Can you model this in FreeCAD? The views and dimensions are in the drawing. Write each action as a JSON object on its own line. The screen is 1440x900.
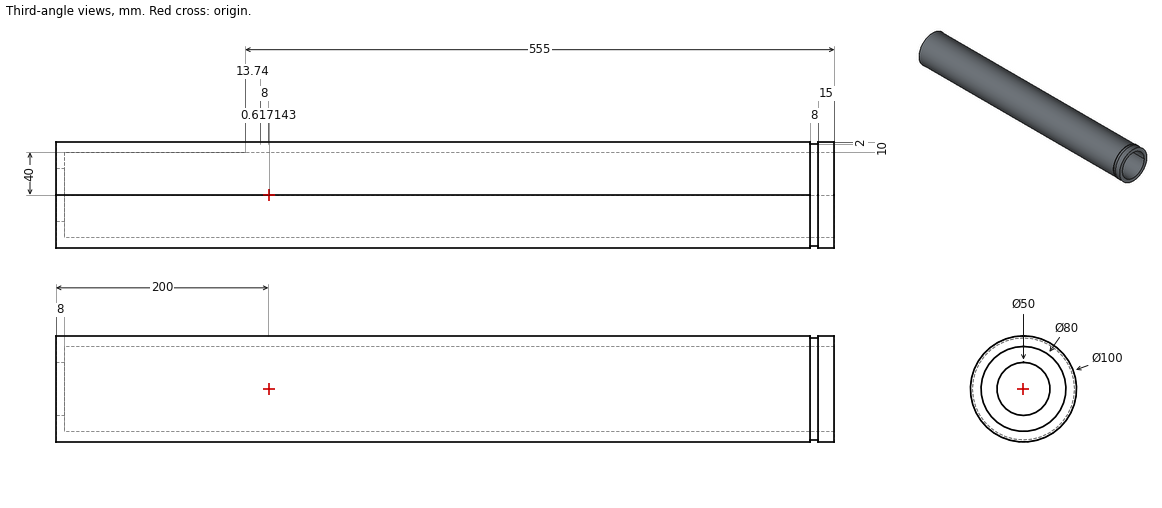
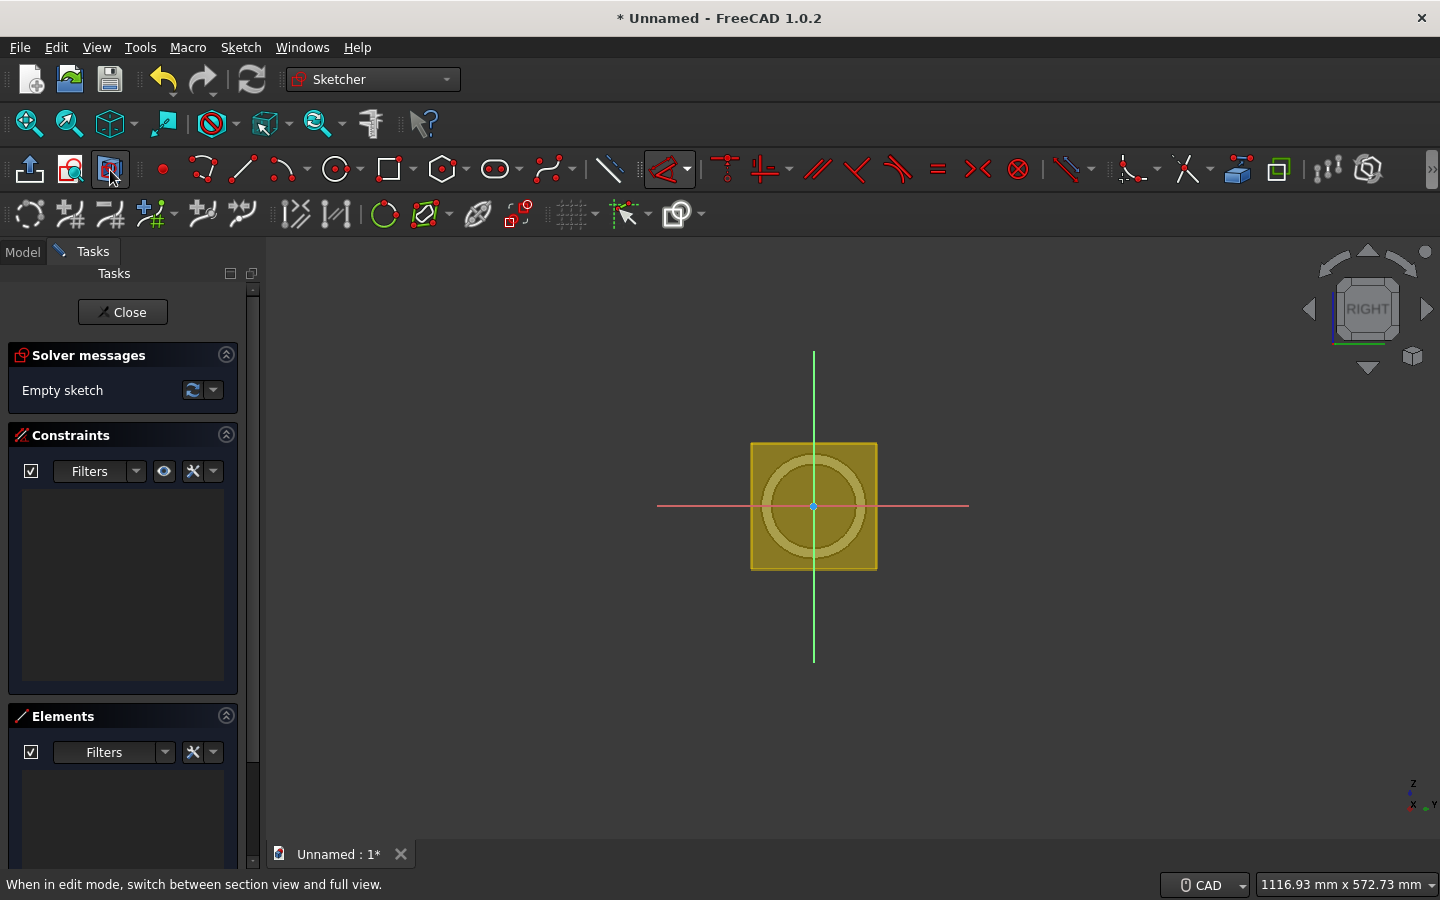
{"action": "scroll", "coordinate": [821, 498], "scroll_direction": "up", "scroll_amount": 8}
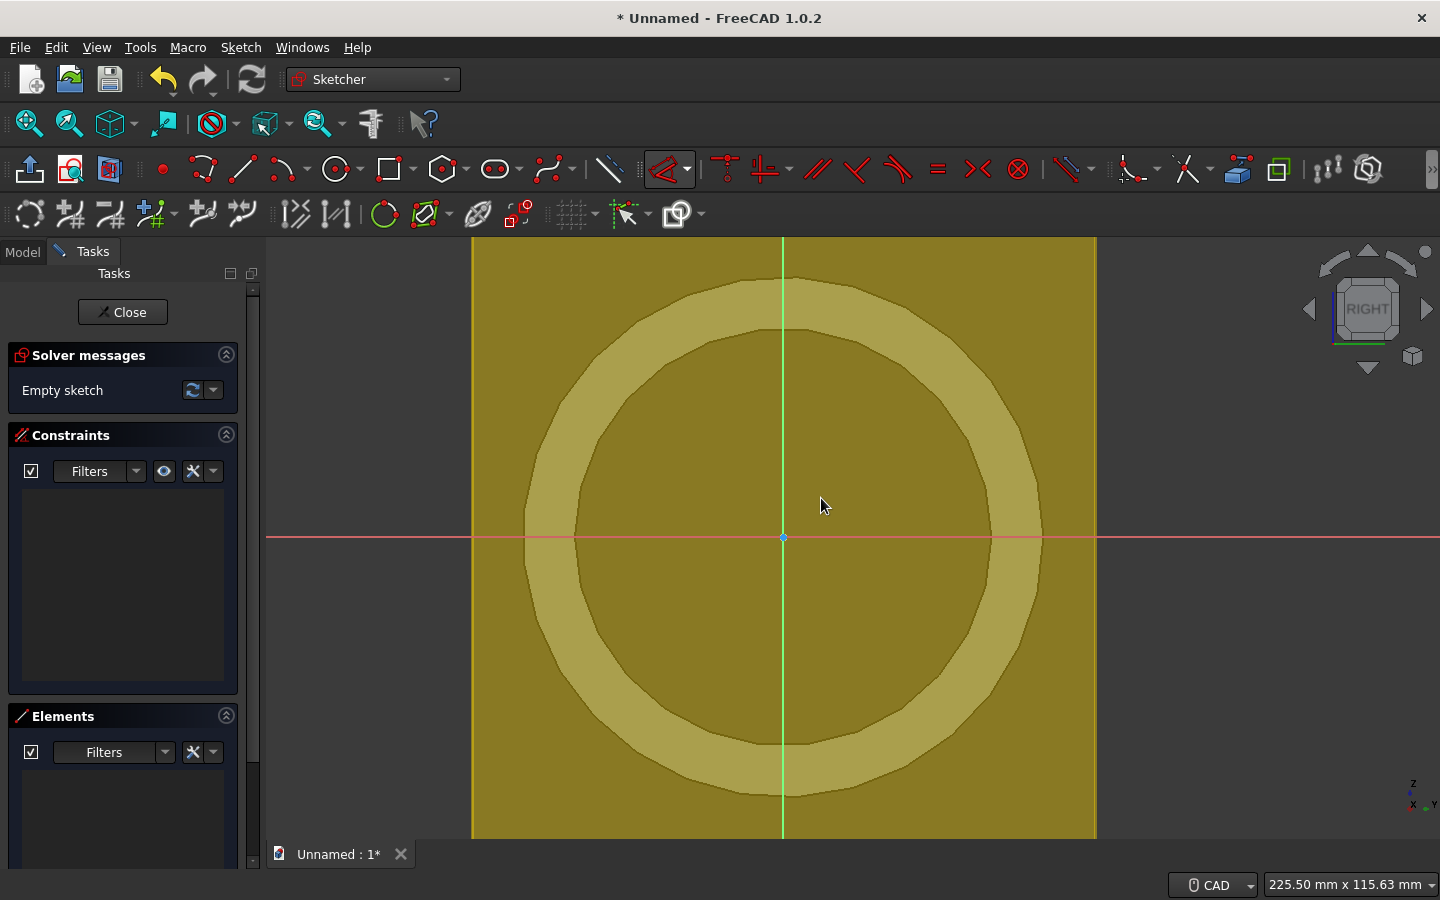
{"action": "key", "text": "g c"}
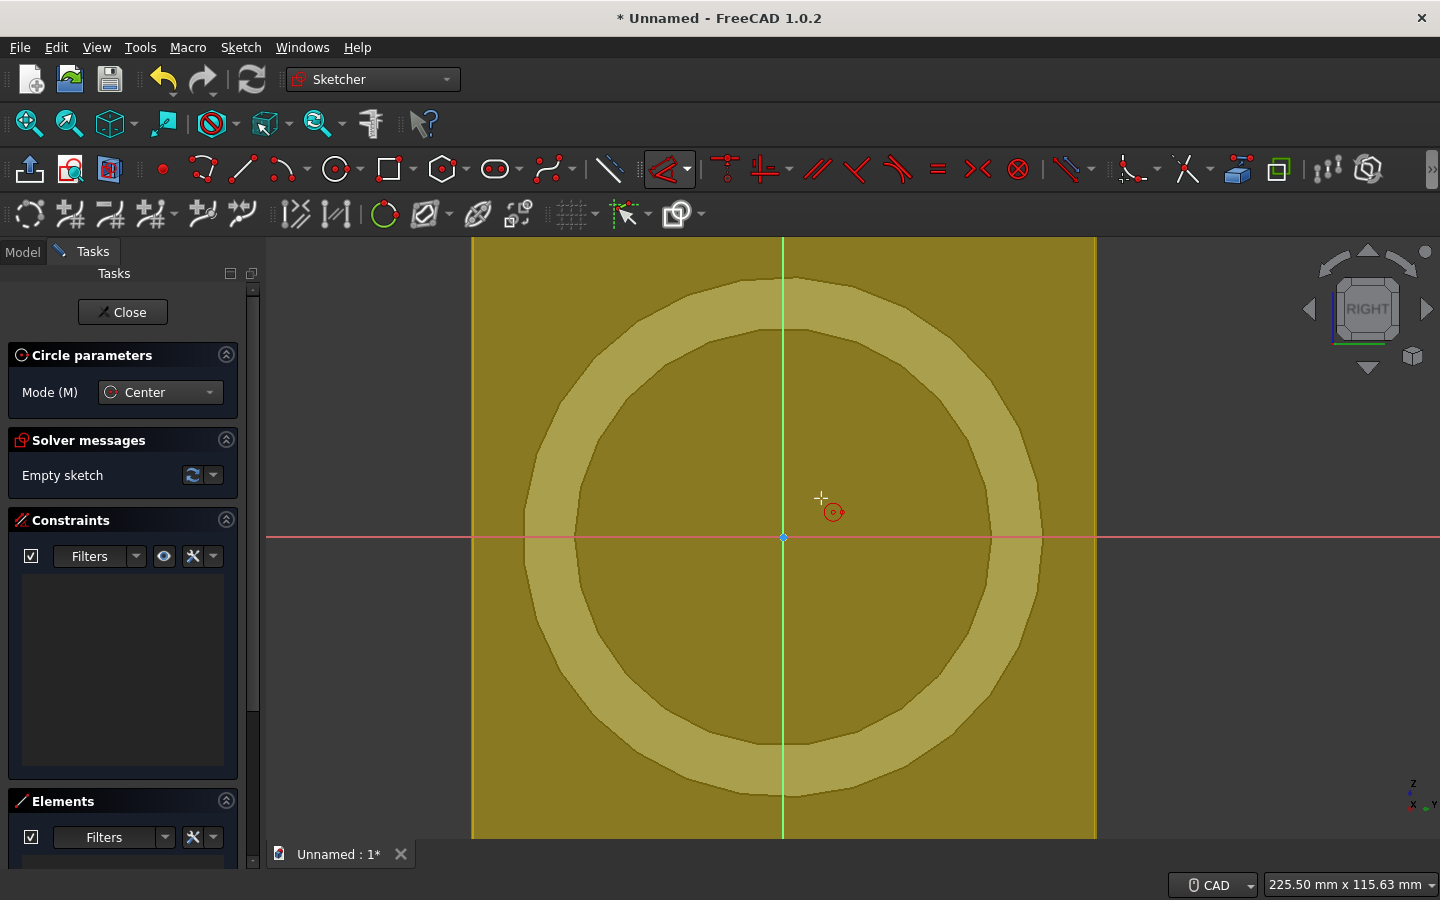
{"action": "left_click", "coordinate": [783, 537]}
{"action": "mouse_move", "coordinate": [930, 390]}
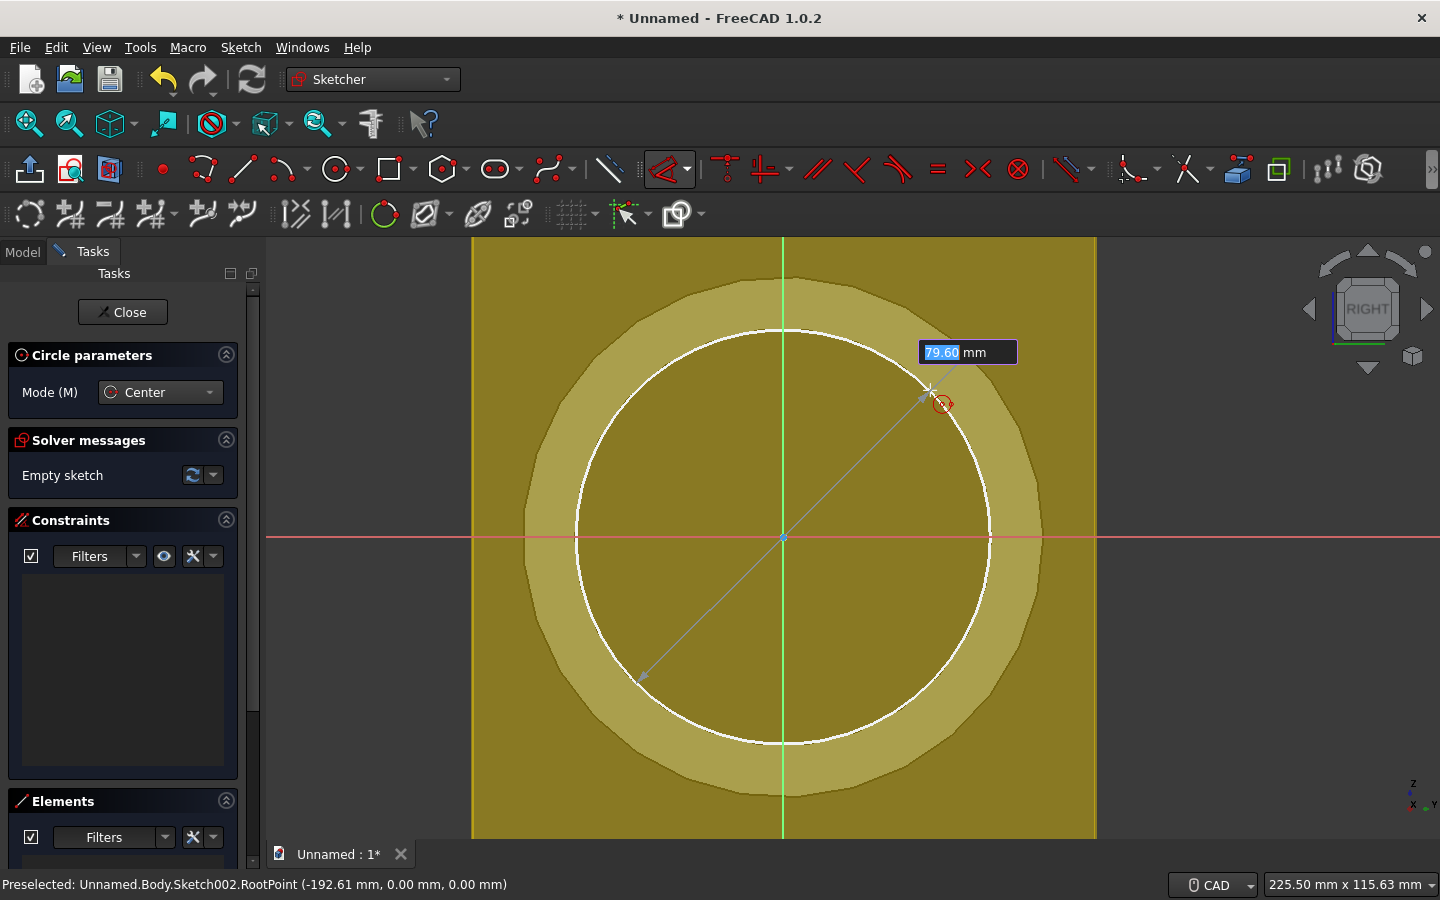
{"action": "type", "text": "80"}
{"action": "key", "text": "Return"}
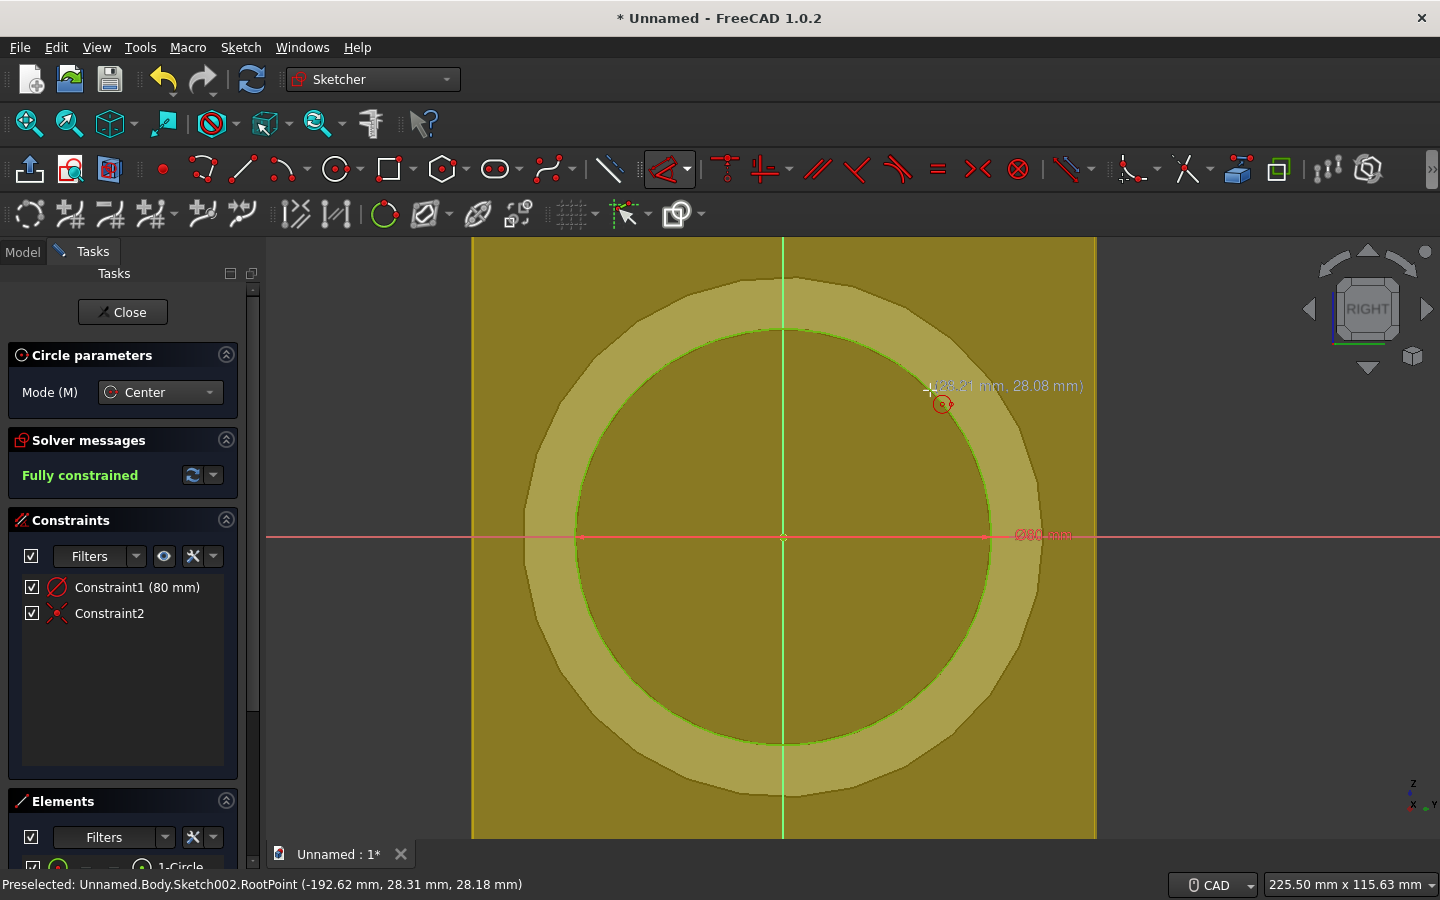
{"action": "left_click", "coordinate": [783, 537]}
{"action": "mouse_move", "coordinate": [875, 445]}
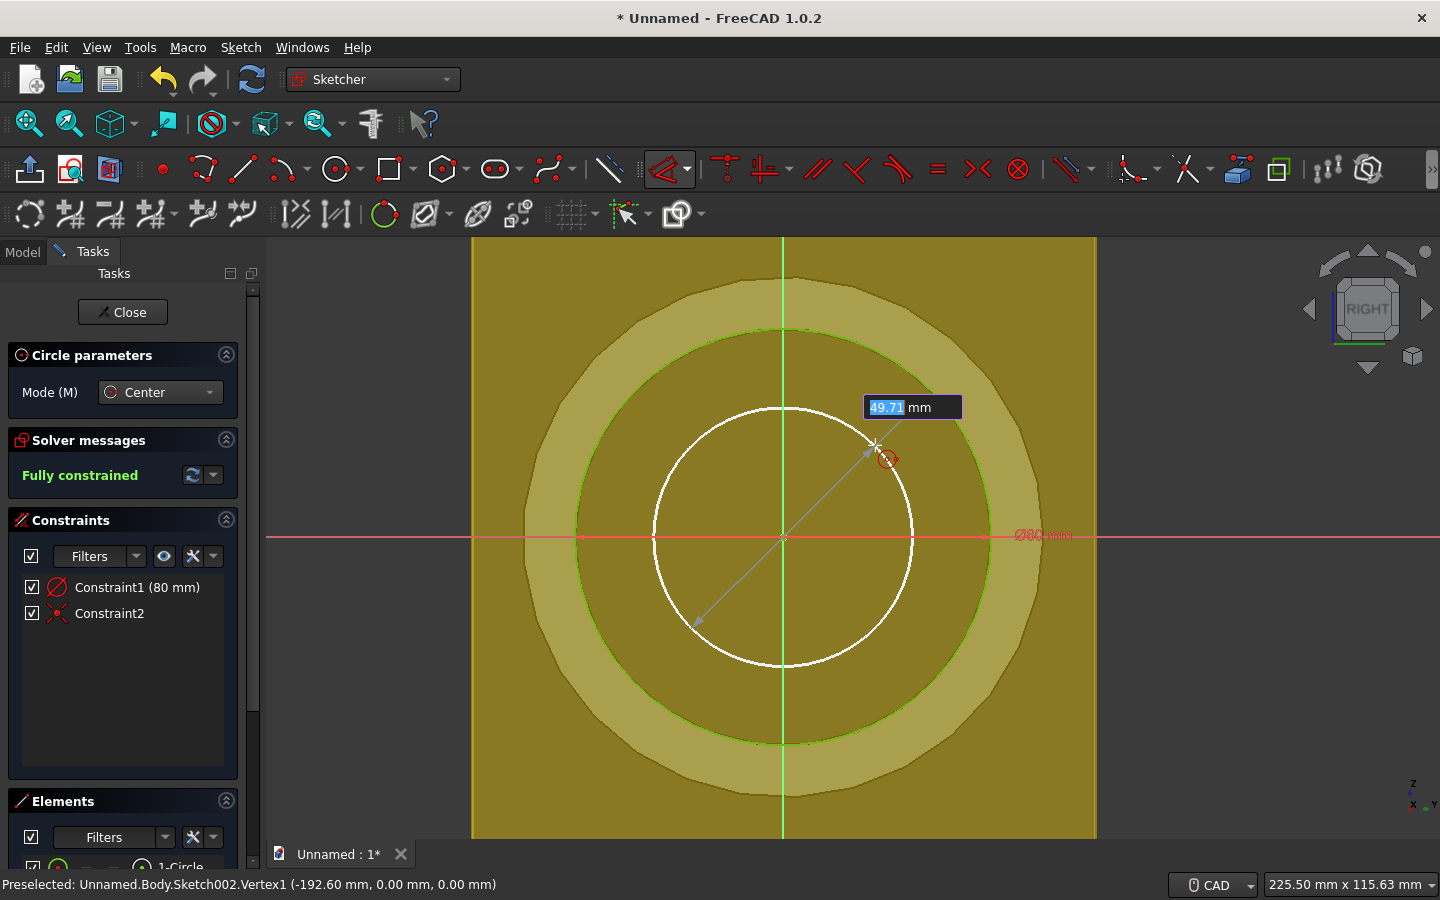
{"action": "type", "text": "50"}
{"action": "key", "text": "Return"}
{"action": "key", "text": "Escape"}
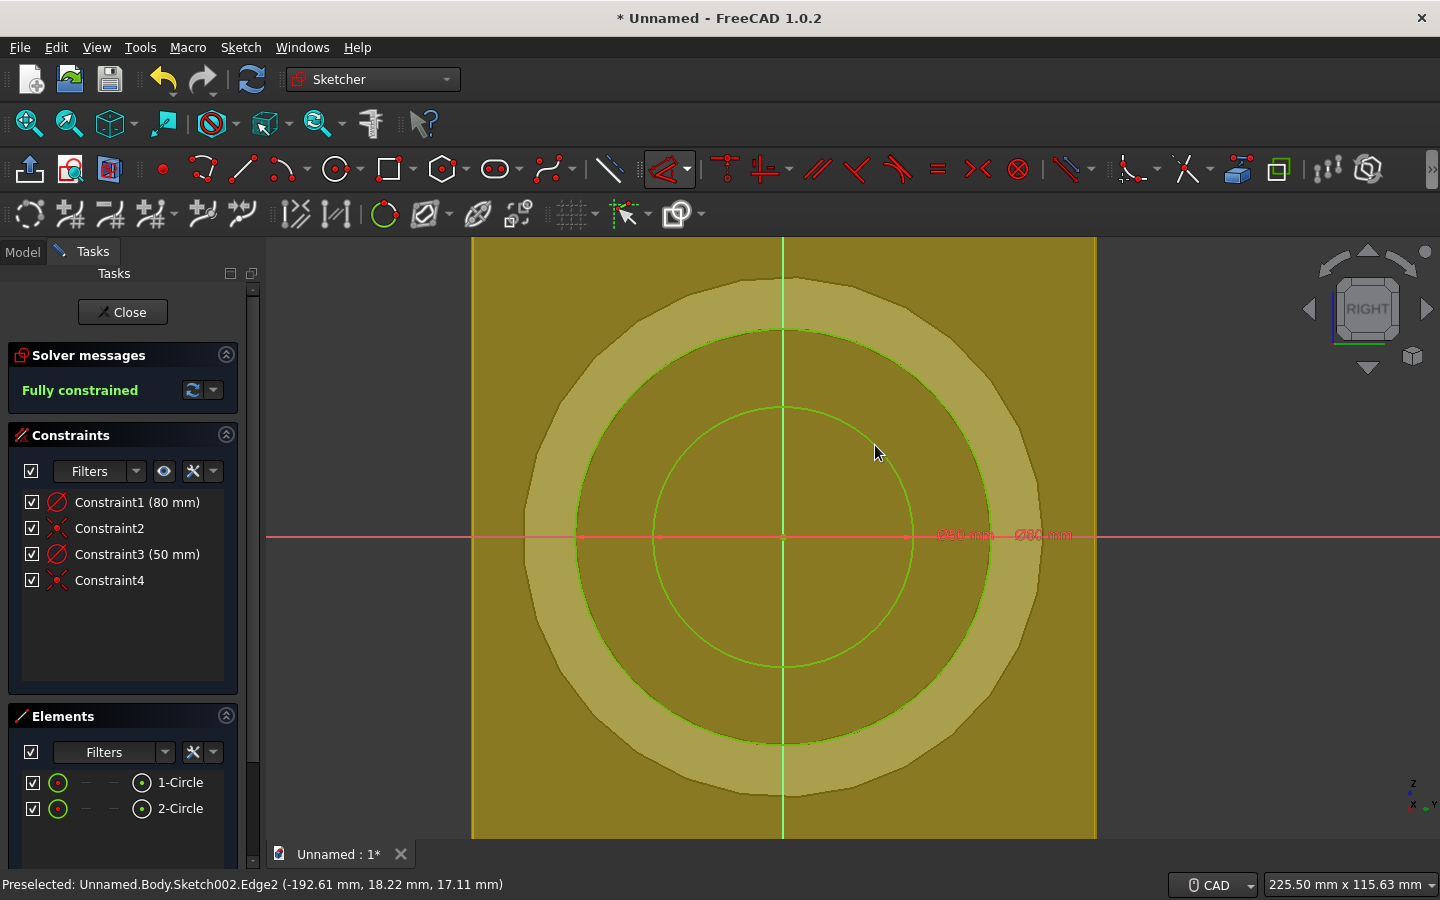
{"action": "left_click", "coordinate": [123, 312]}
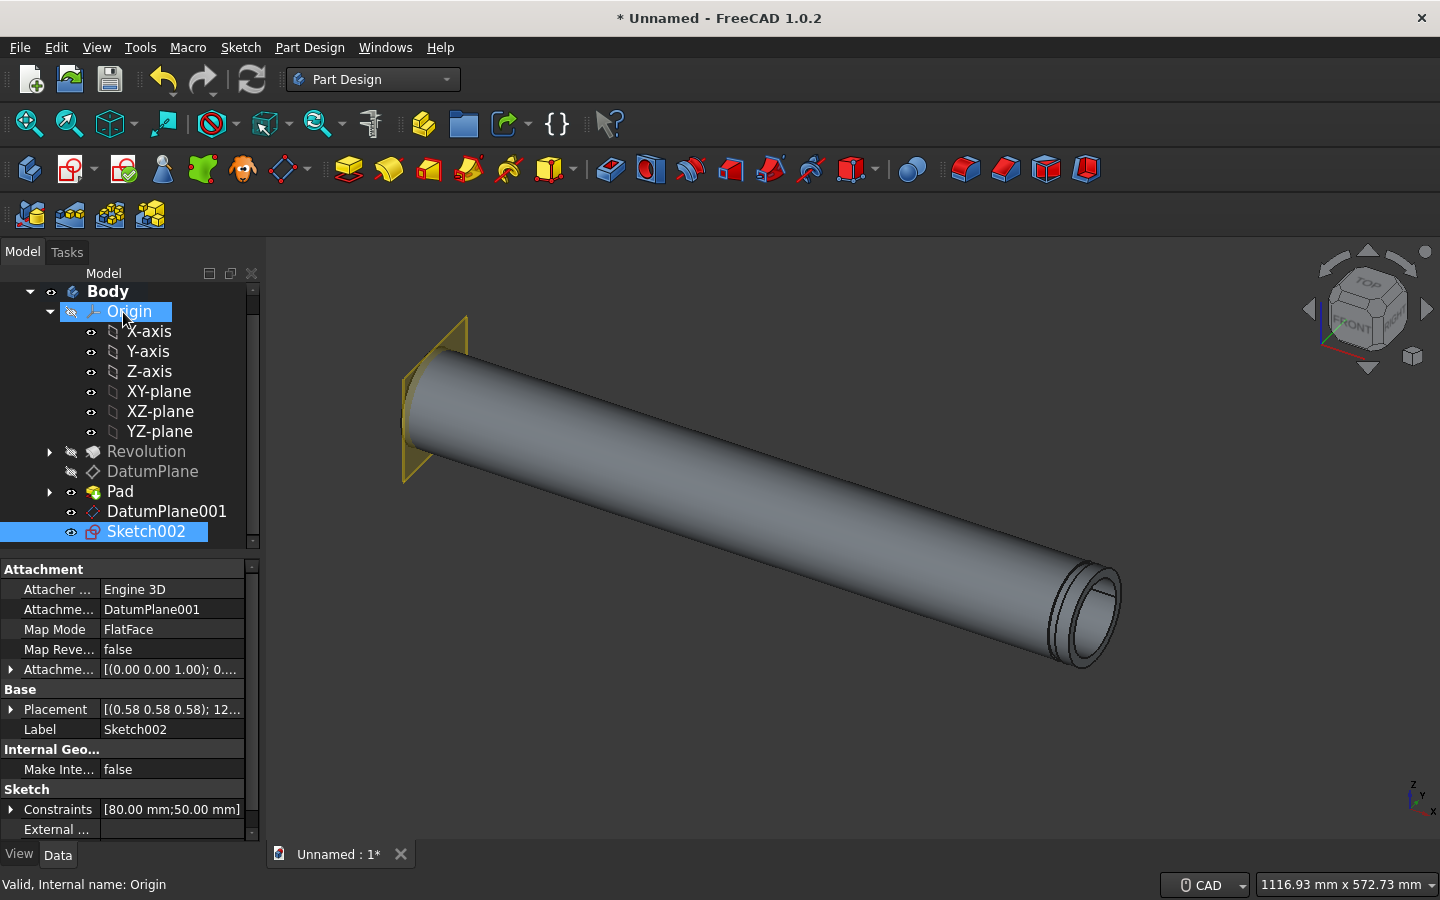
{"action": "left_click", "coordinate": [350, 170]}